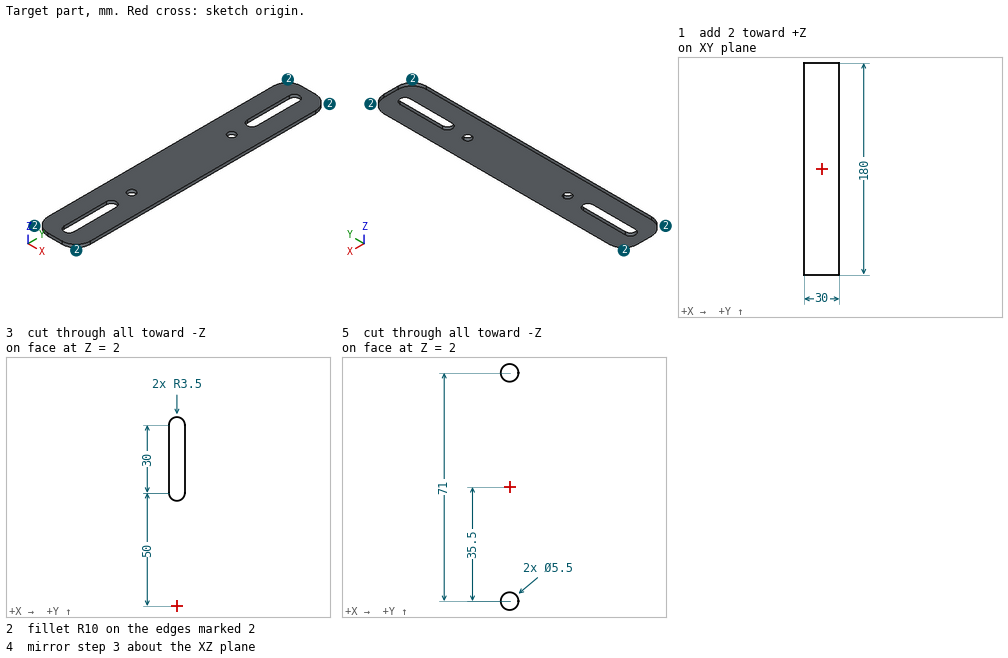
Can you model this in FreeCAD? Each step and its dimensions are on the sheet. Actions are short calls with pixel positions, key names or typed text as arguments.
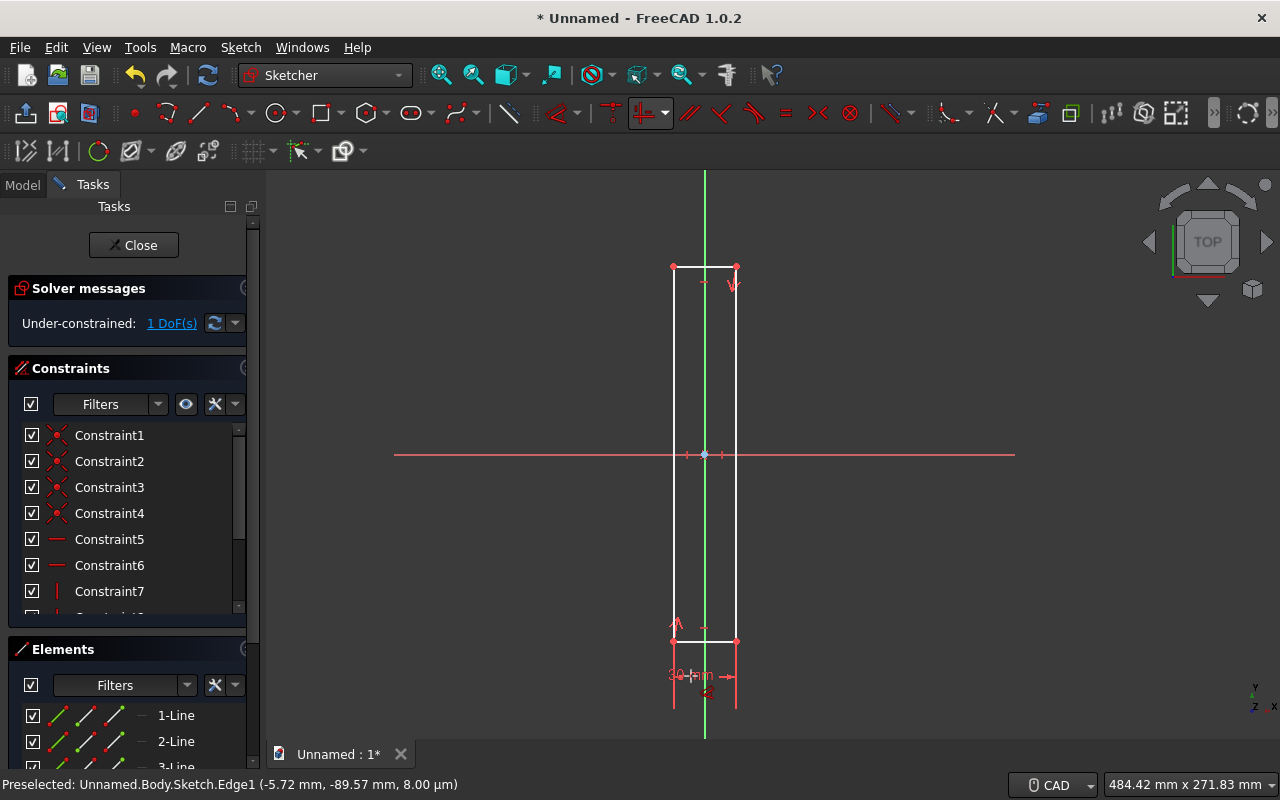
click(736, 529)
click(770, 368)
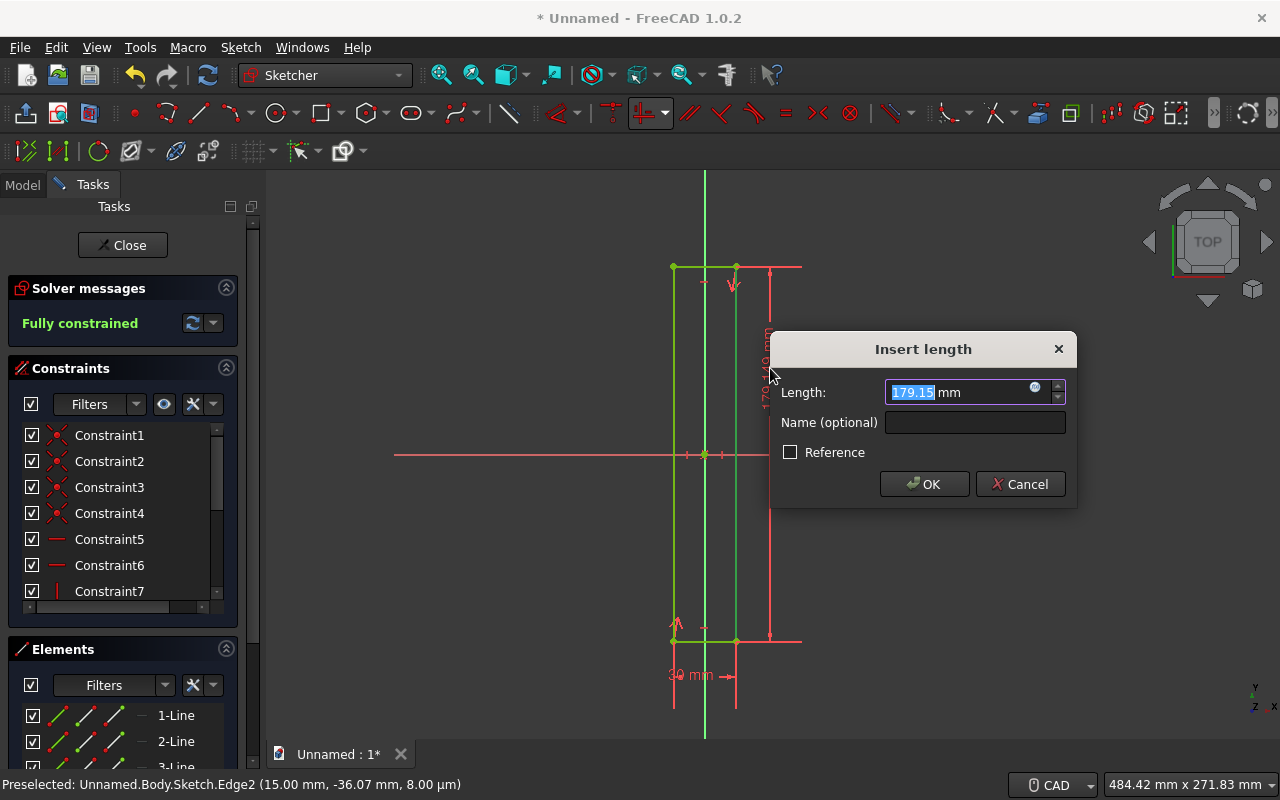
text(180)
key(Return)
key(Escape)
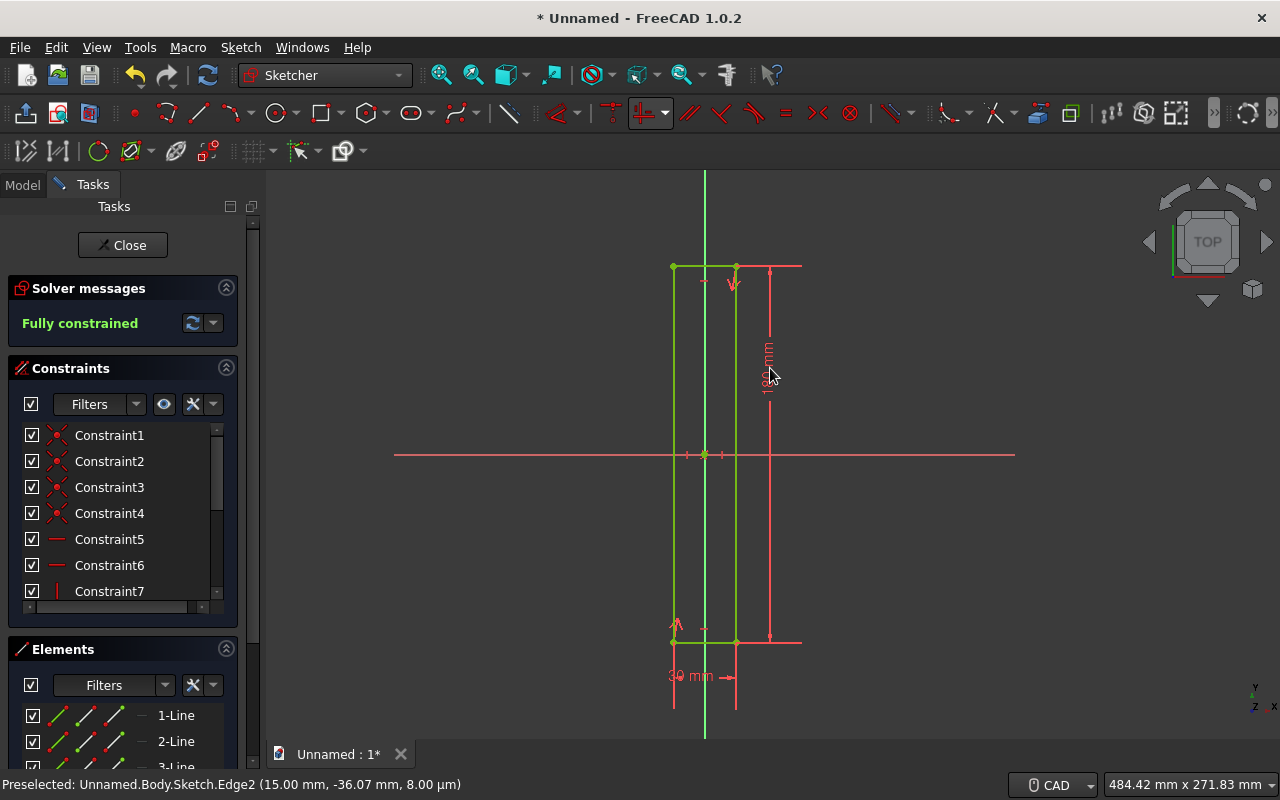
click(123, 245)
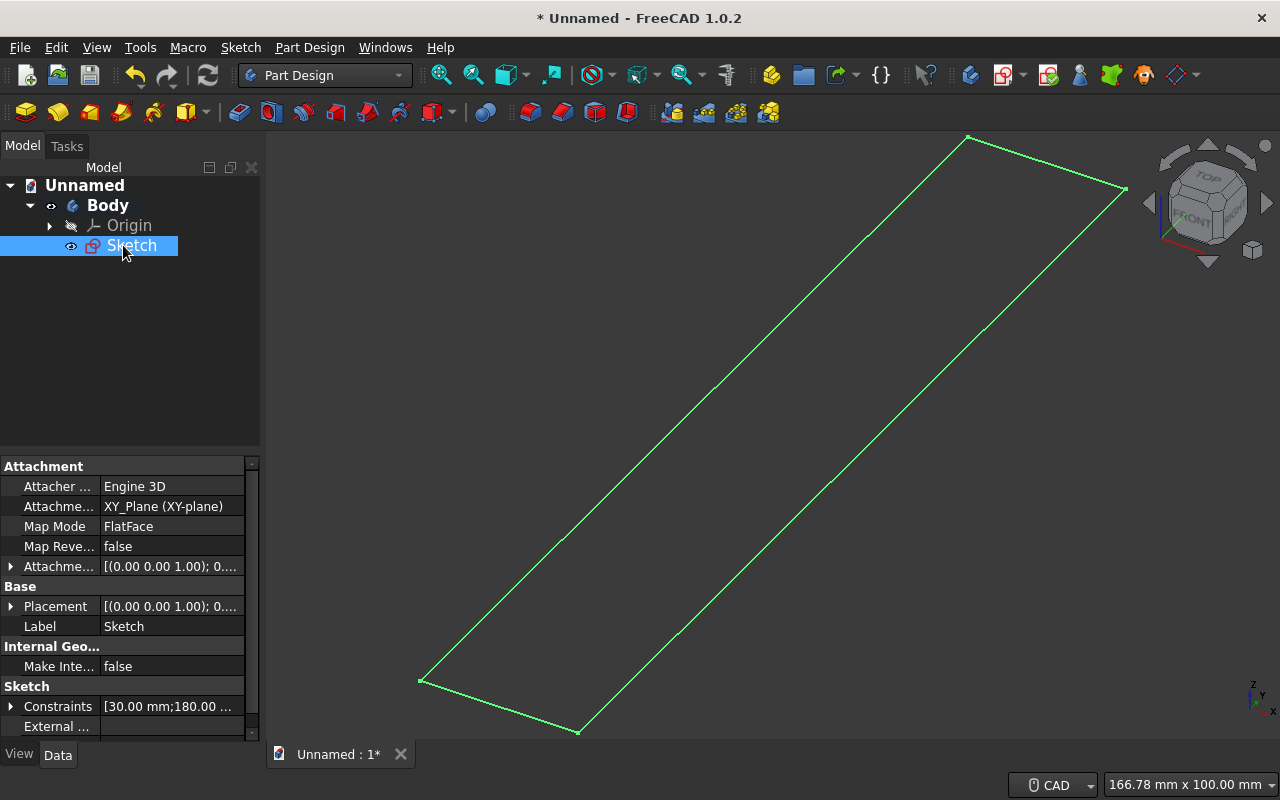
click(26, 112)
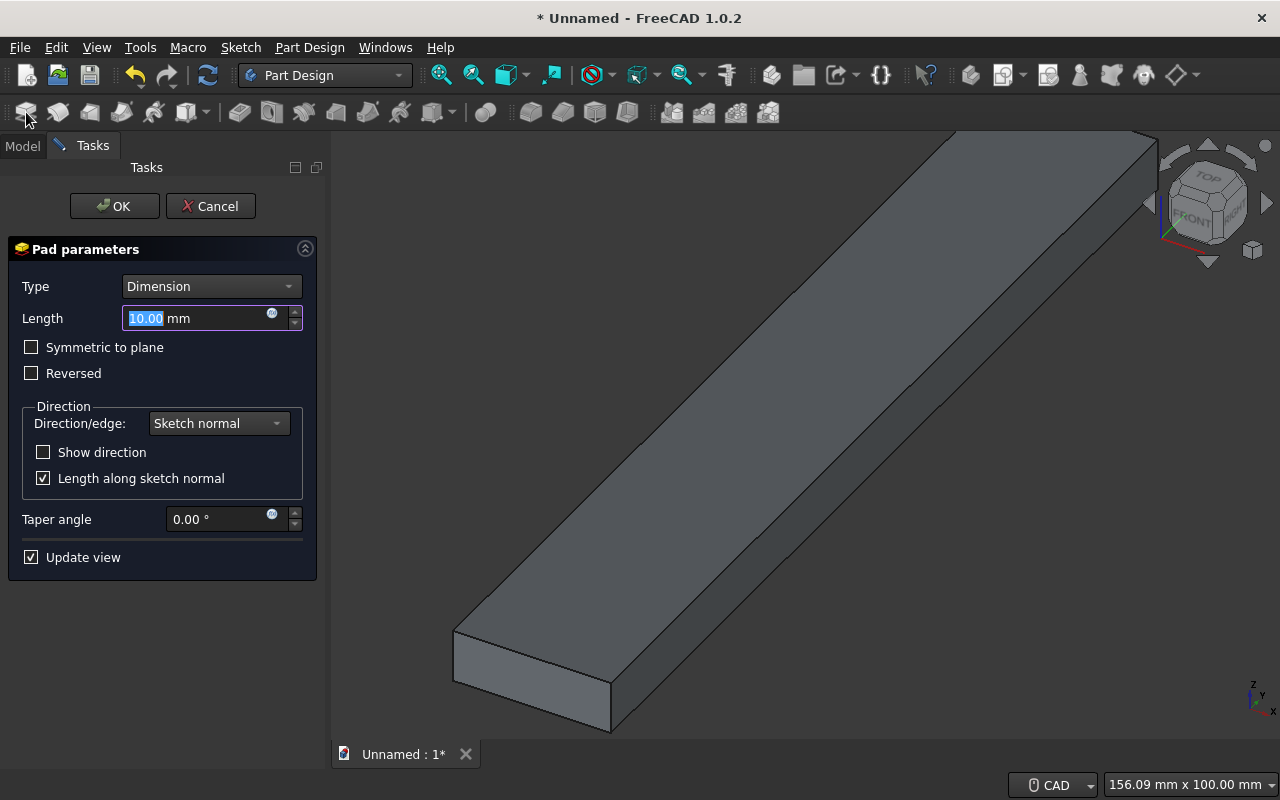
text(2)
key(Tab)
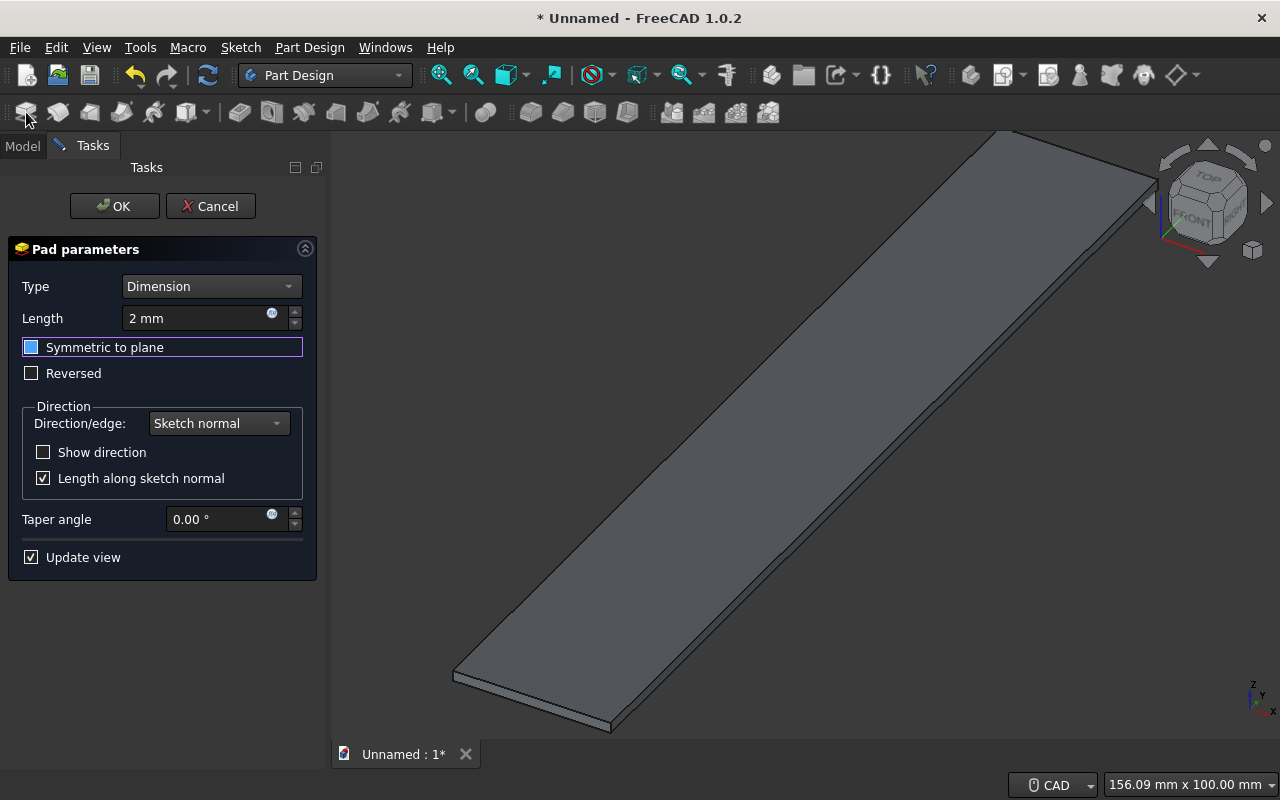
click(115, 206)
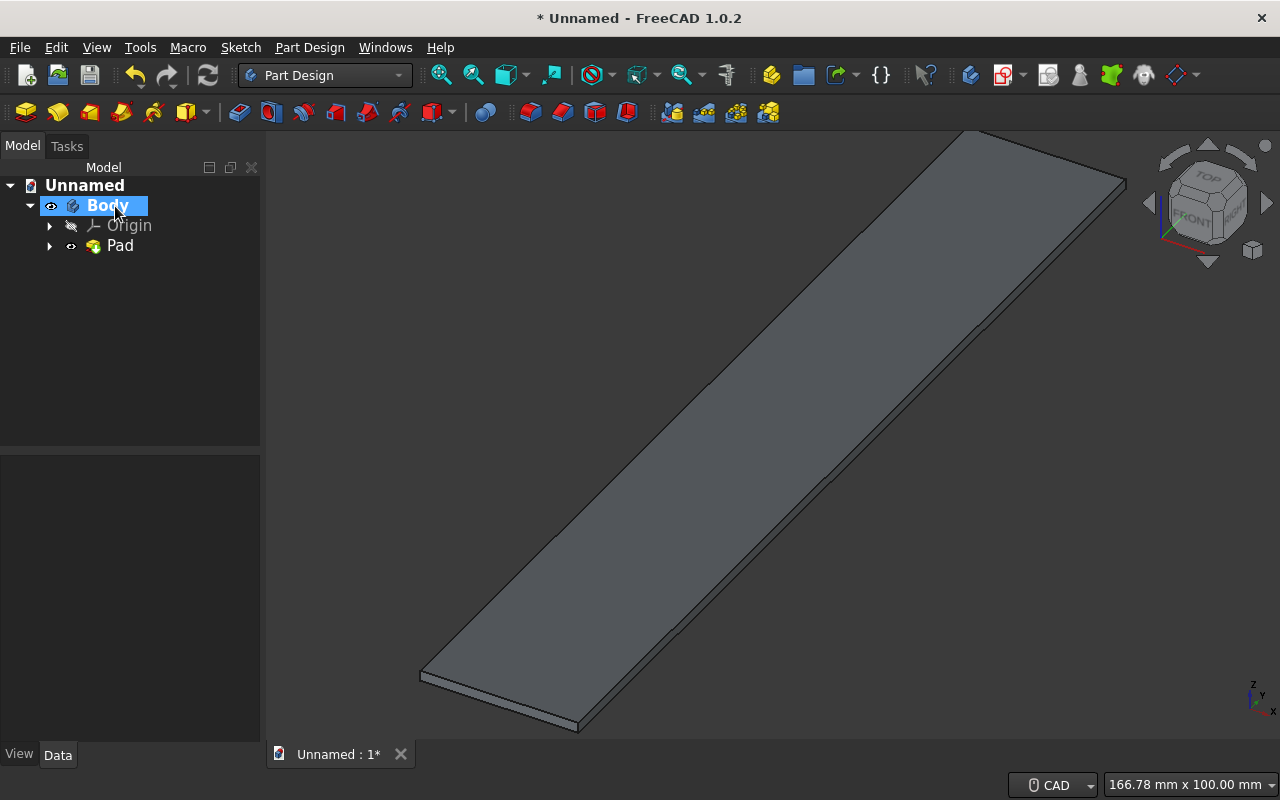
key(v)
key(f)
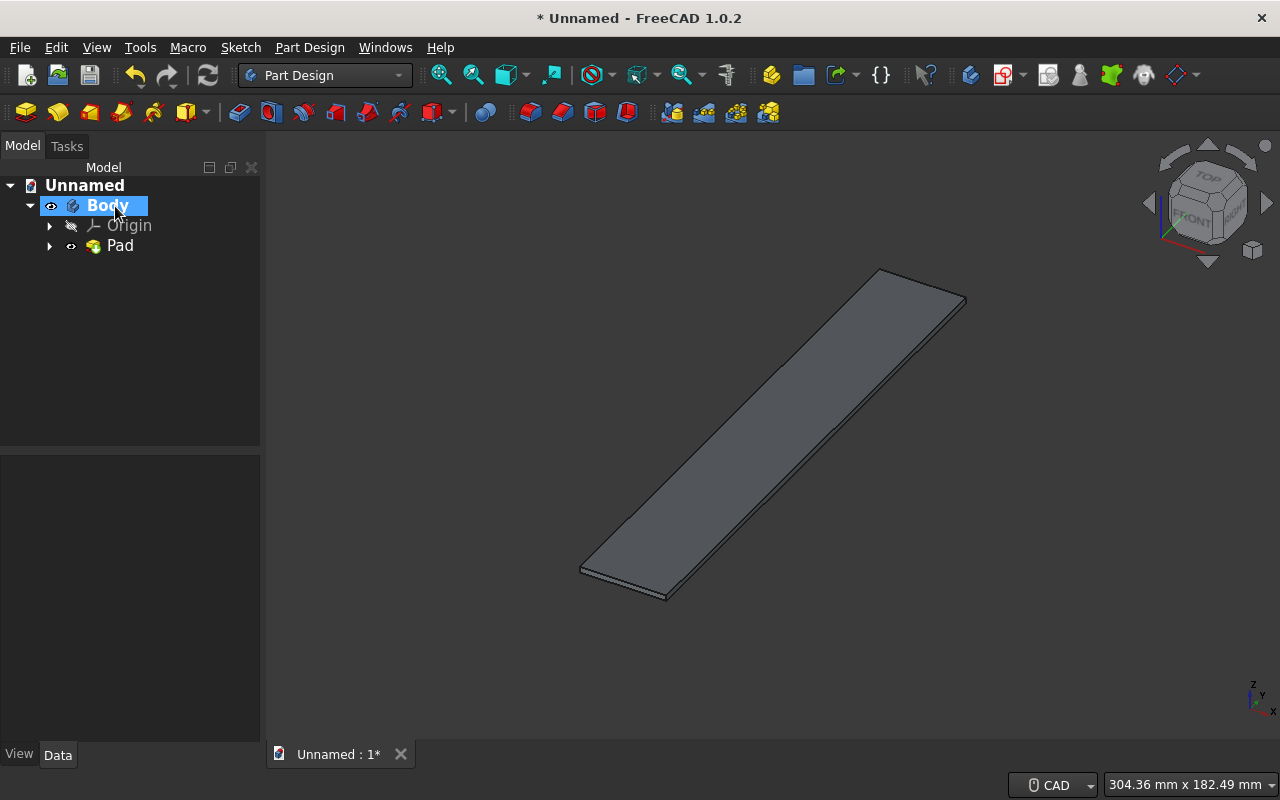
scroll(880, 271, up, 9)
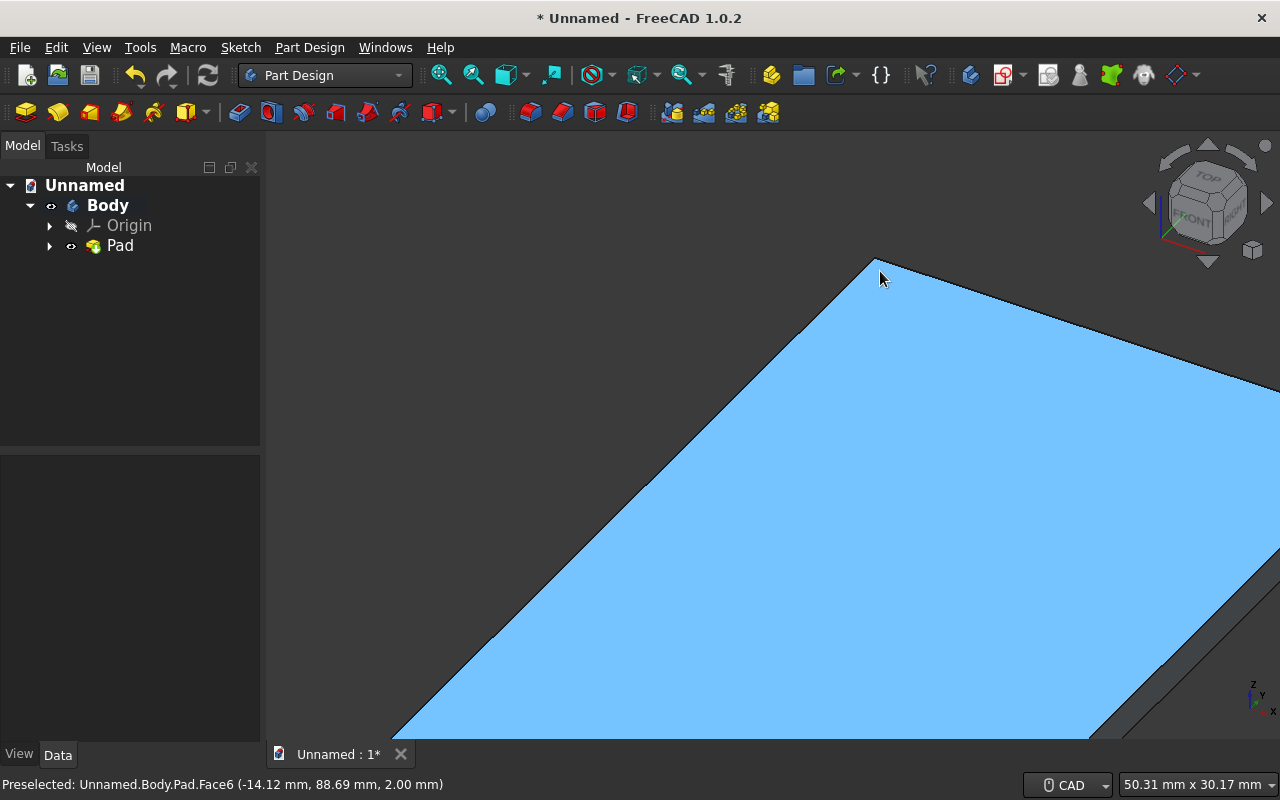
key(v)
key(f)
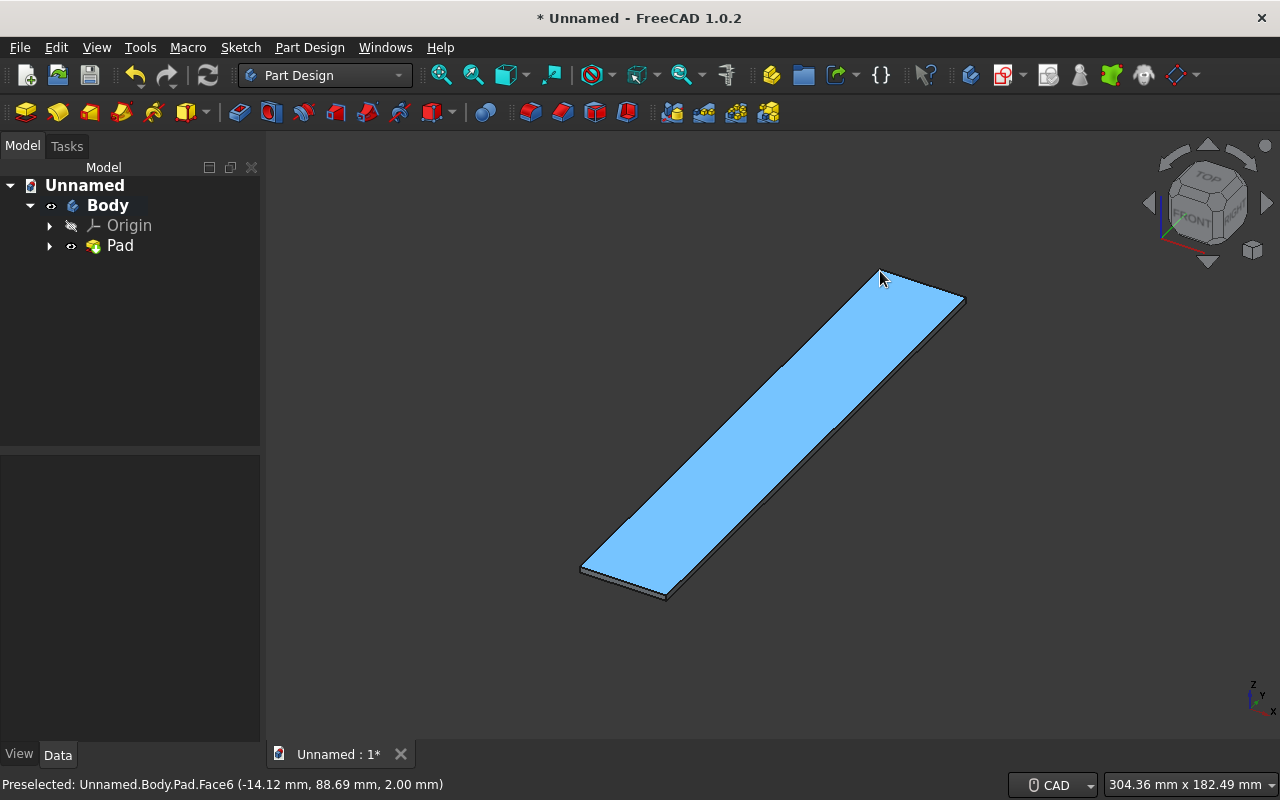
key(0)